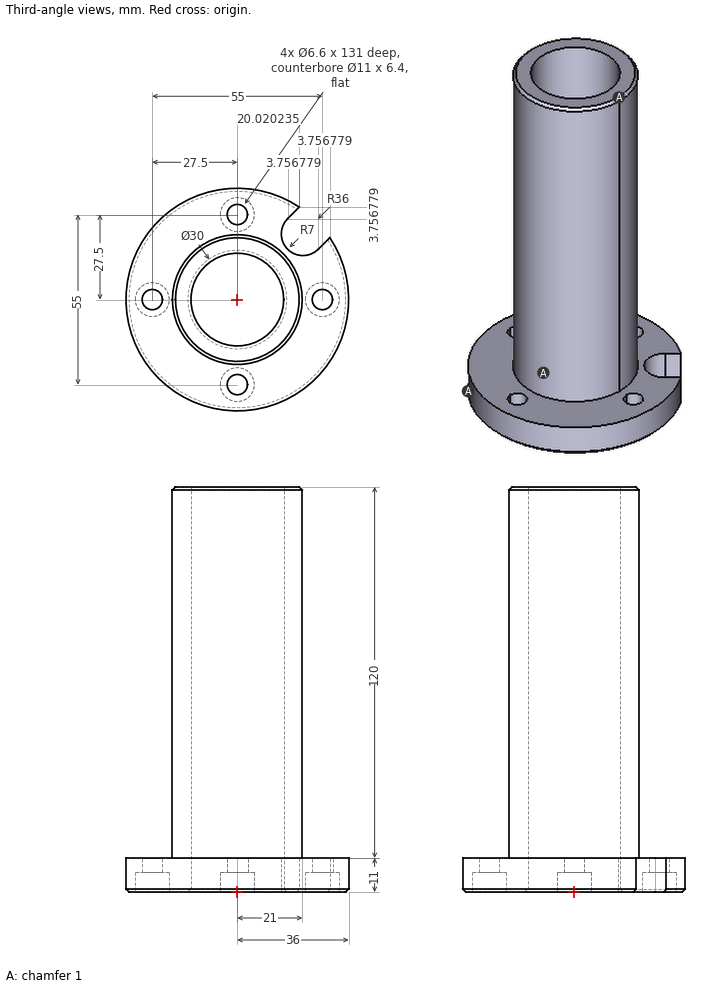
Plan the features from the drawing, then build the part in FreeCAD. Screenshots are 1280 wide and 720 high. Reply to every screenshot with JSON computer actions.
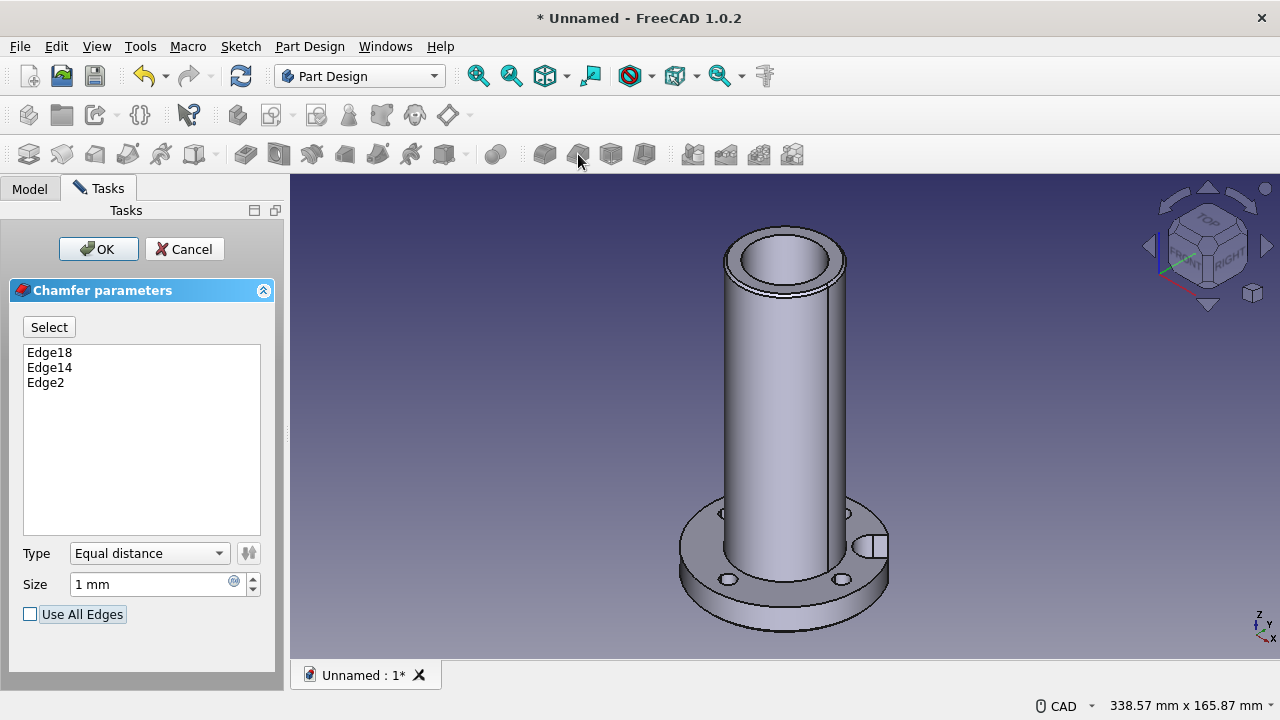
{"action": "left_click", "coordinate": [99, 249]}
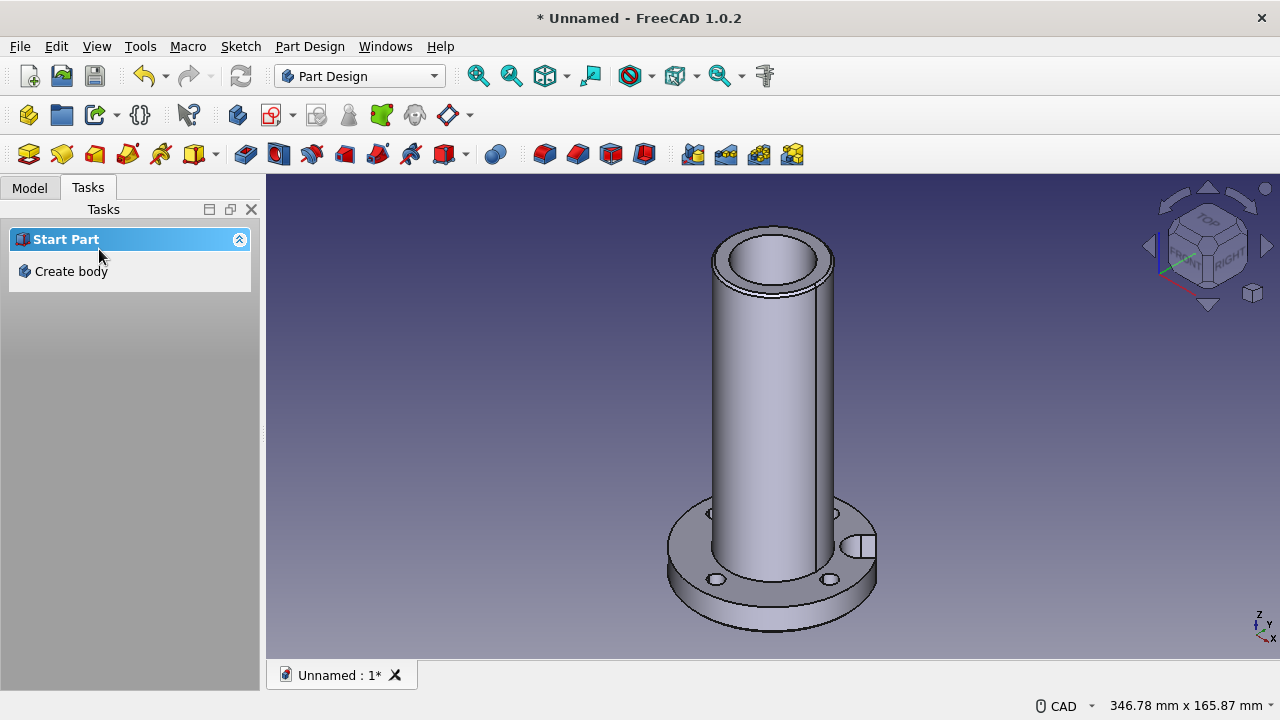
{"action": "left_click", "coordinate": [479, 76]}